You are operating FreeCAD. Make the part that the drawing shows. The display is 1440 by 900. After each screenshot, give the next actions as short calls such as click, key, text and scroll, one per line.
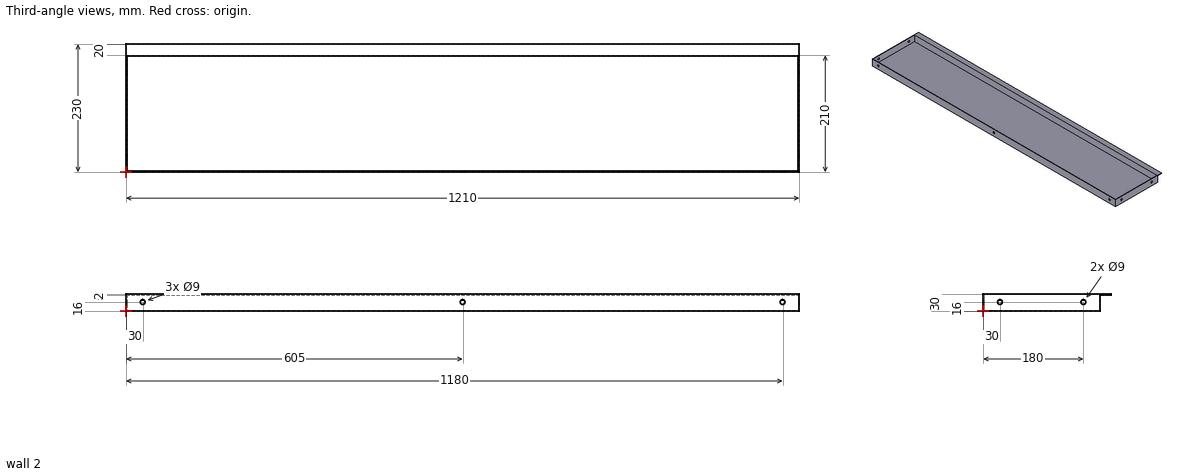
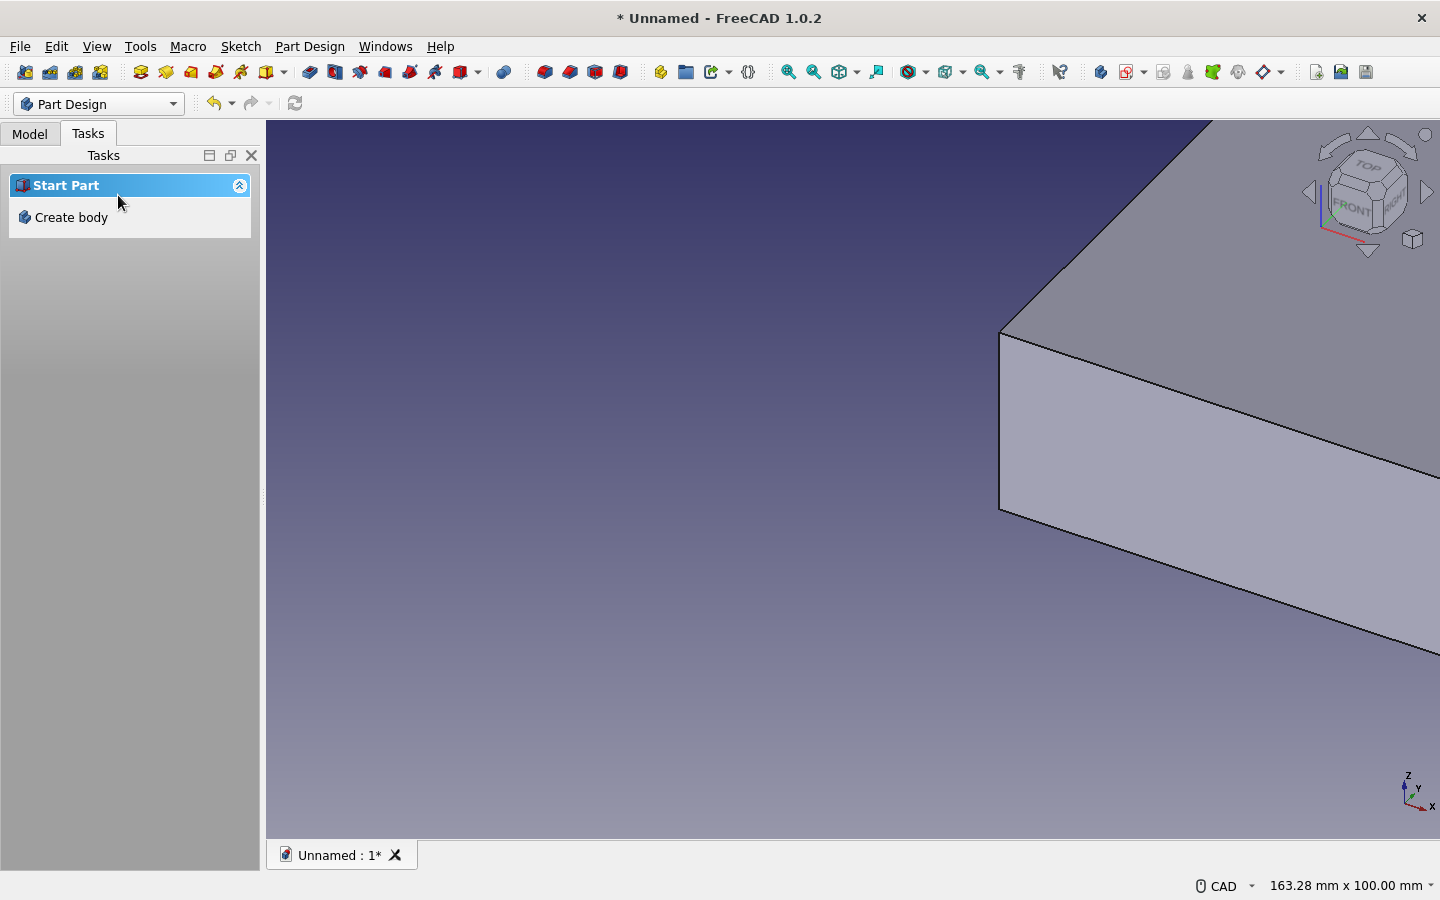
click(789, 72)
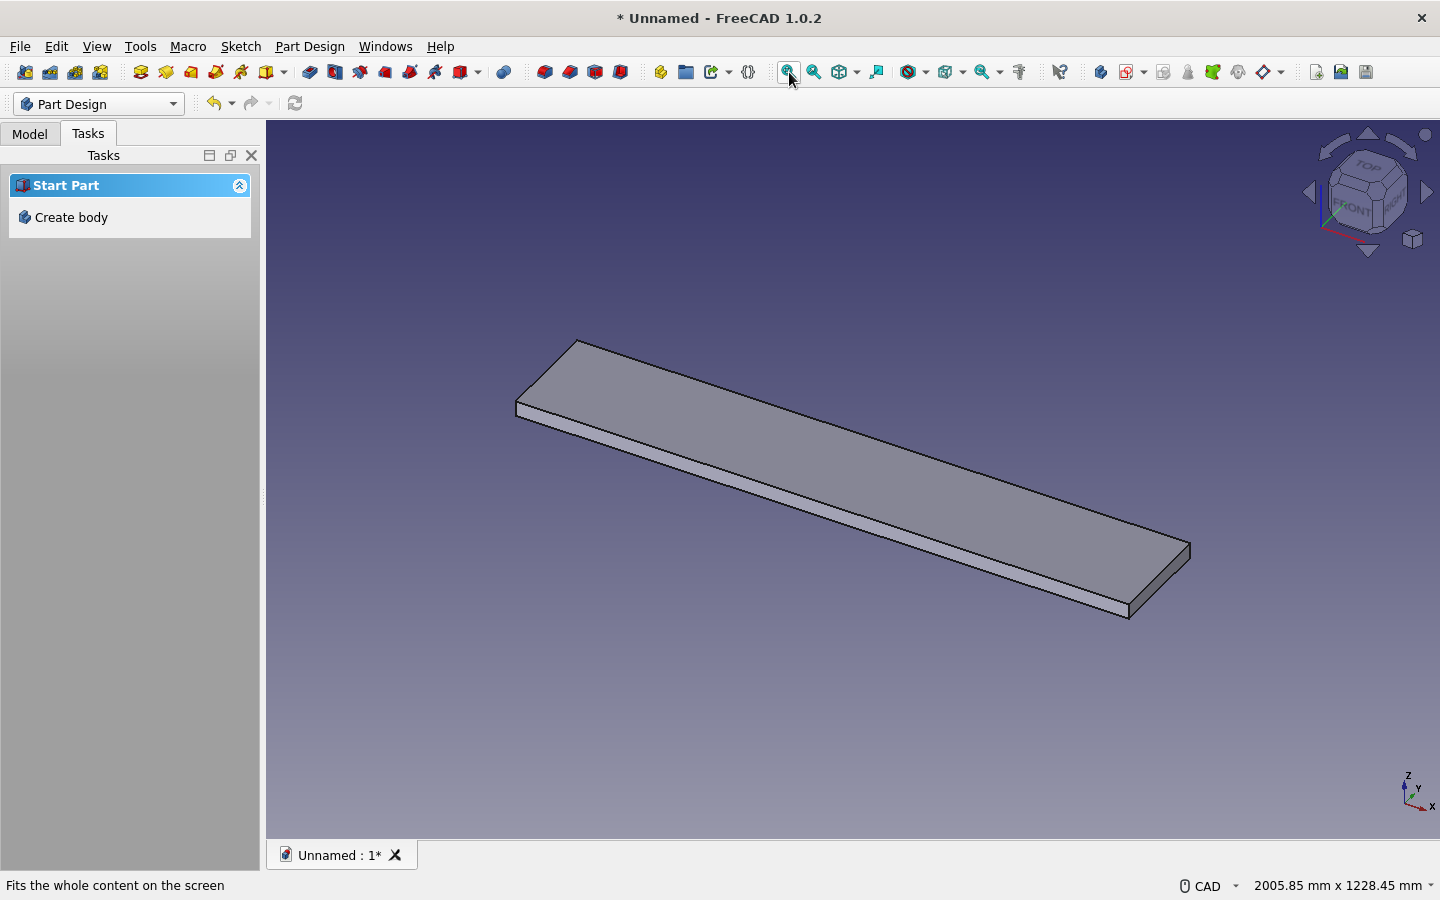
click(1028, 529)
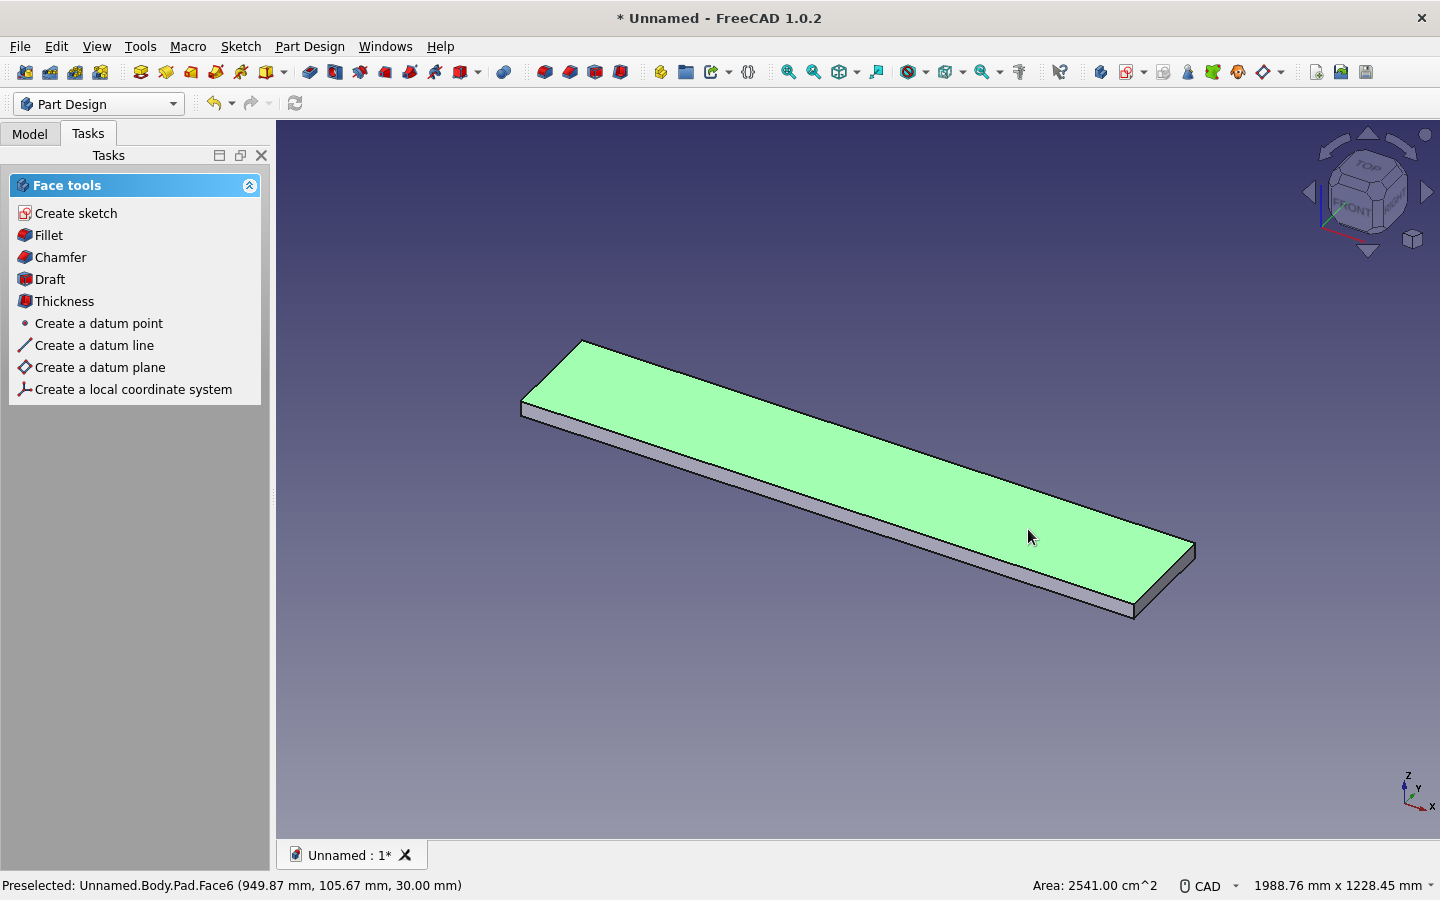
click(620, 72)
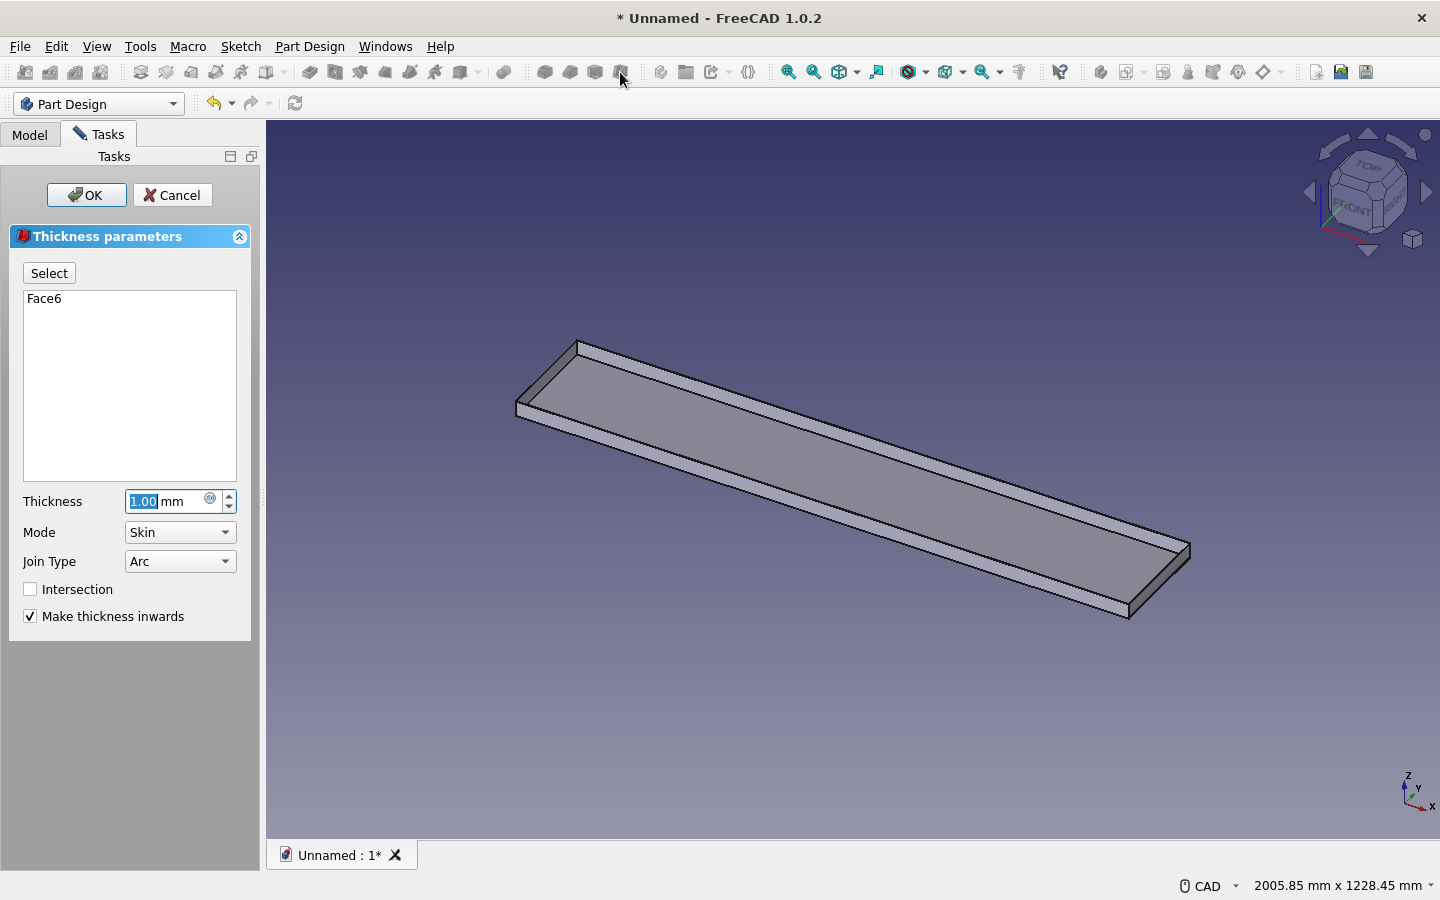
text(2)
key(Tab)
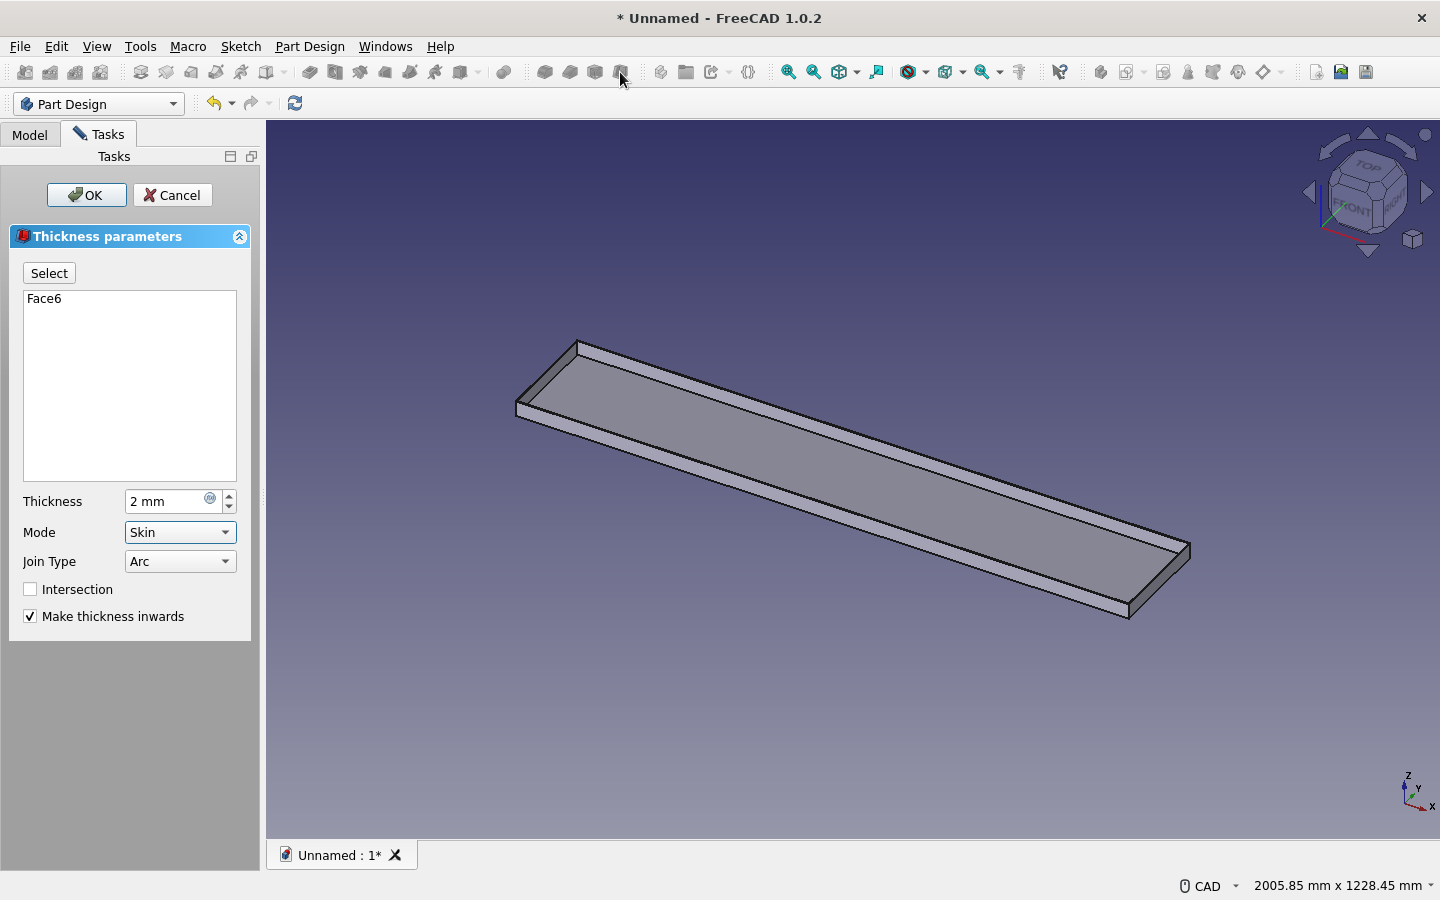
click(181, 562)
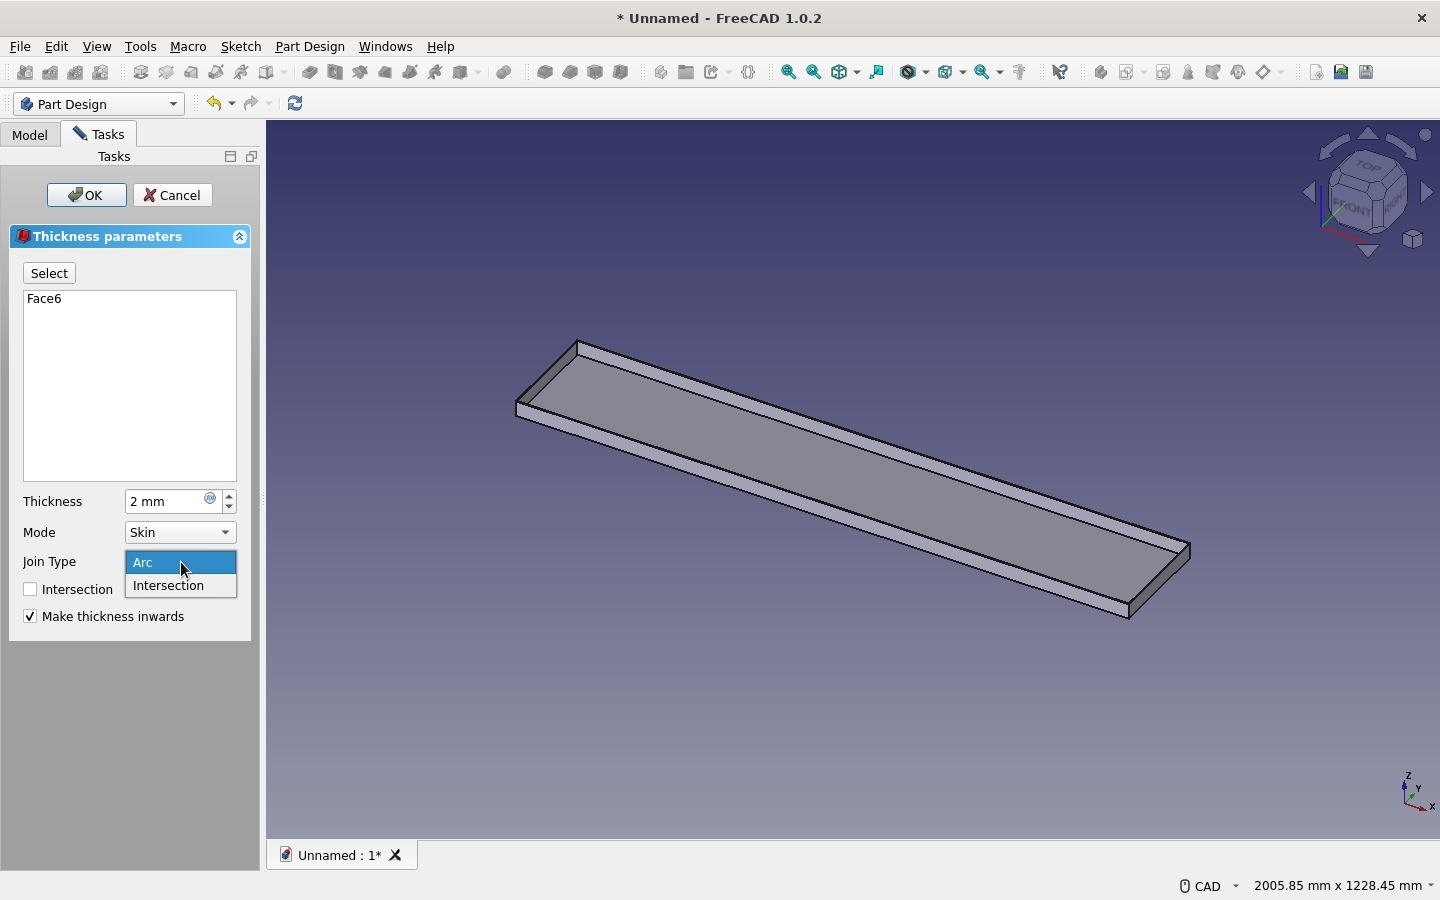
click(179, 586)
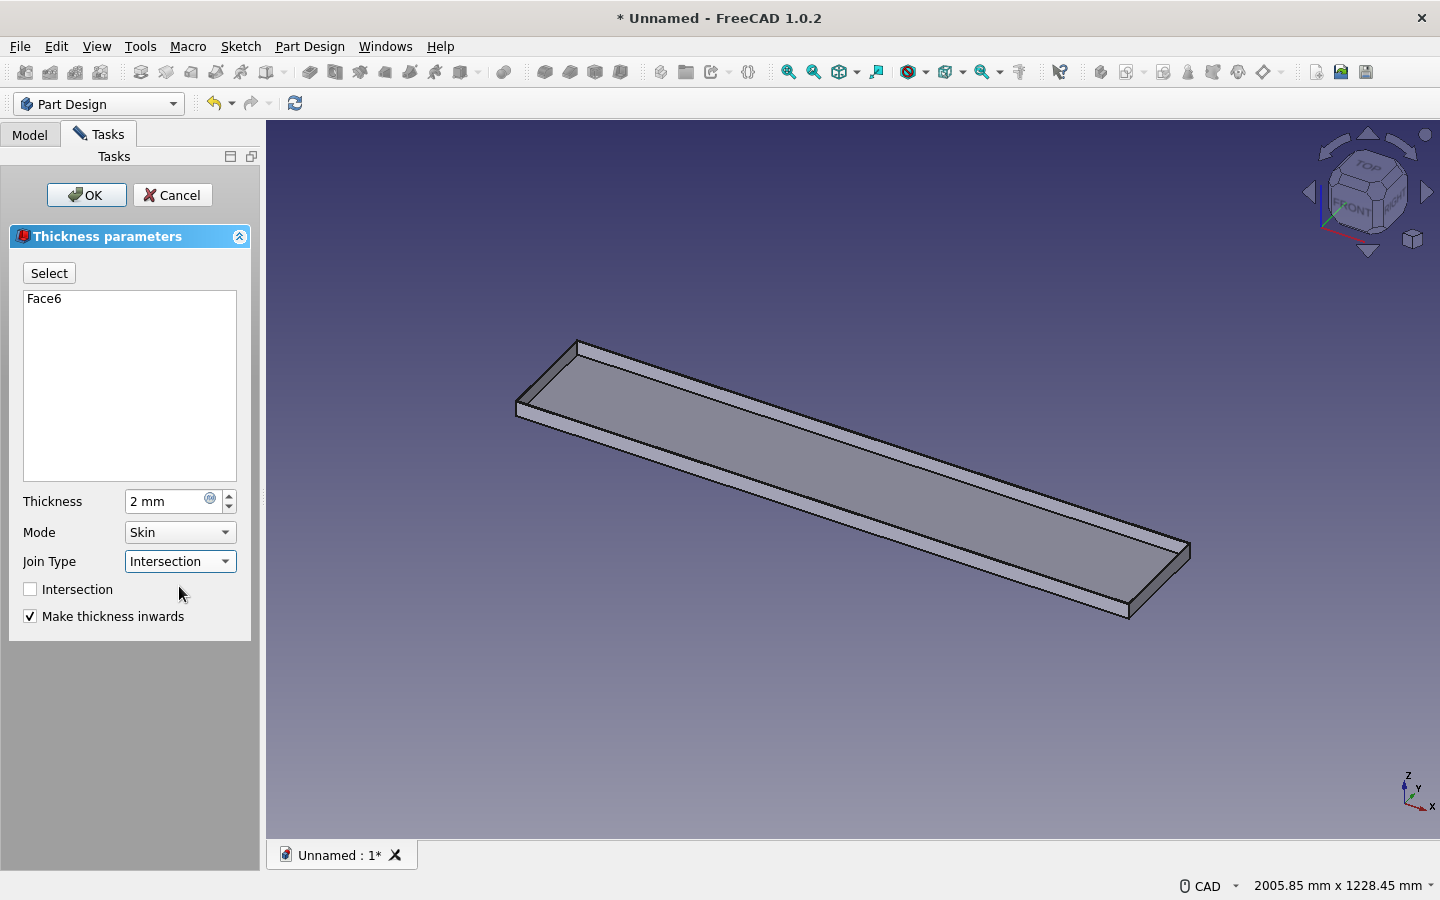
click(87, 195)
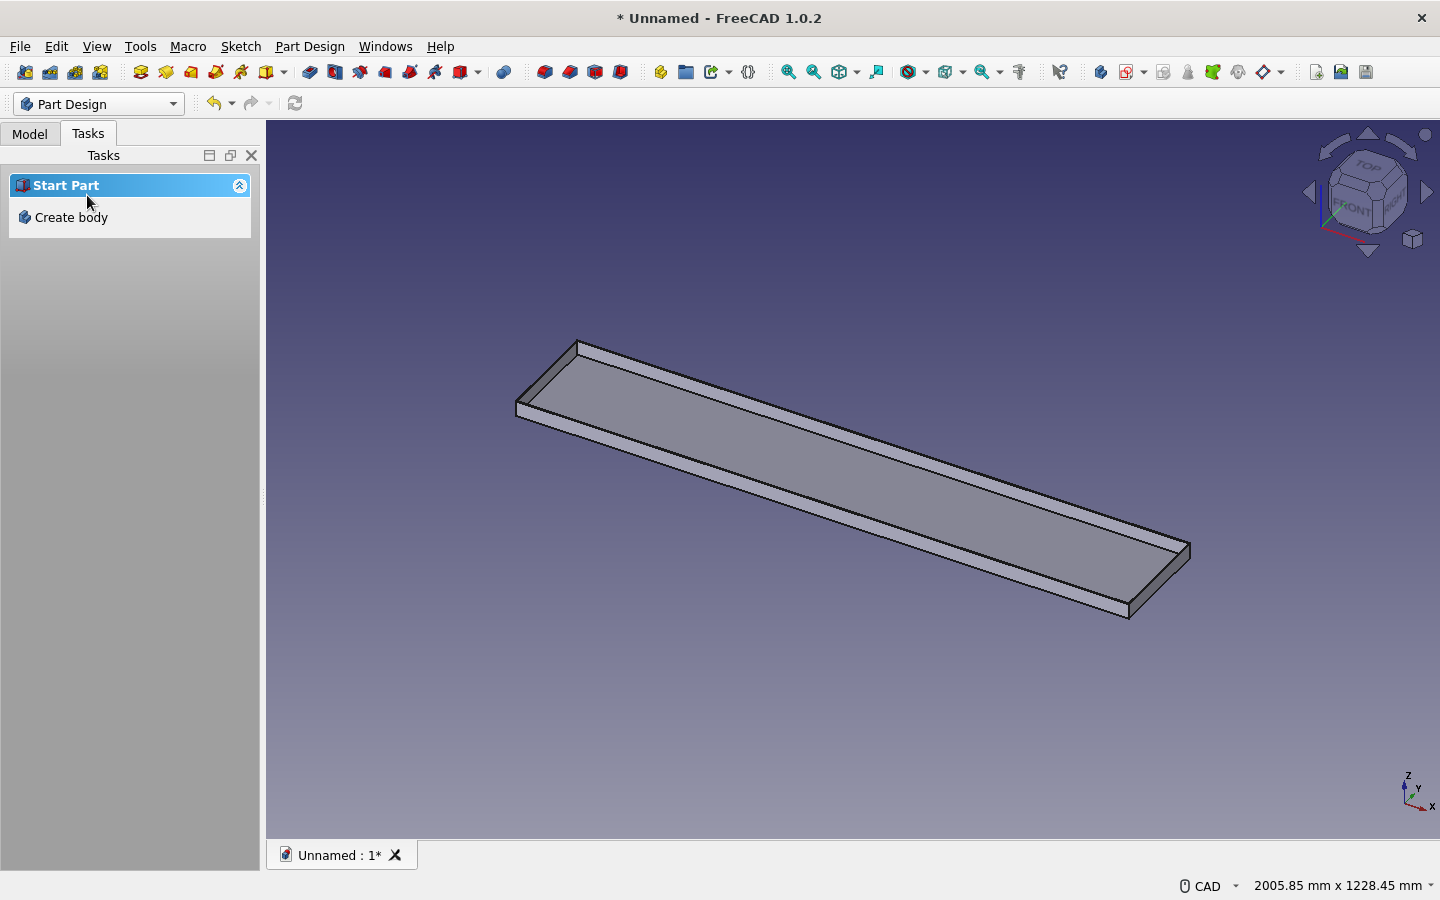
scroll(1169, 563, up, 15)